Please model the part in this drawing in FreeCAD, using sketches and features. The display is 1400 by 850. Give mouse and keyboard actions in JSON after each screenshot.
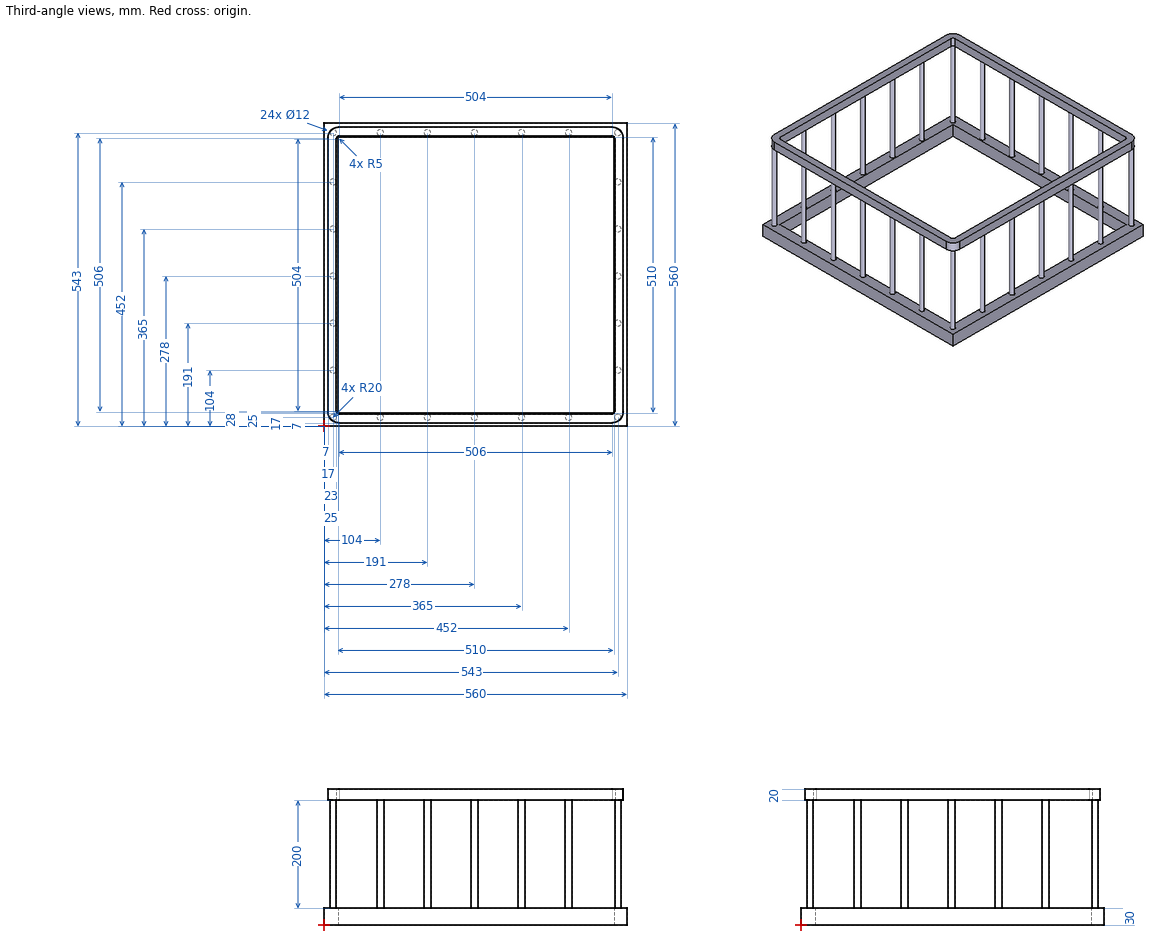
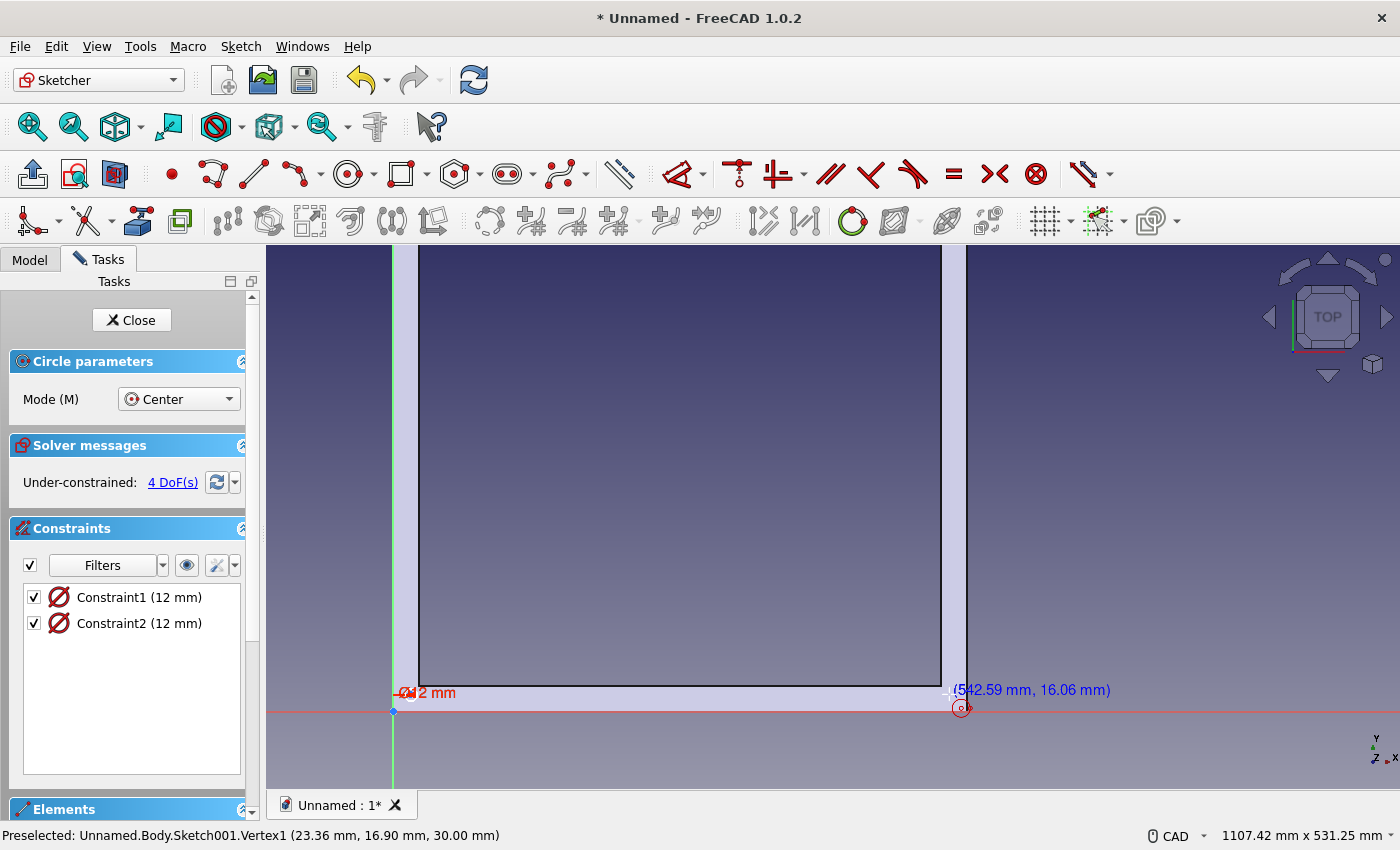
{"action": "left_click", "coordinate": [949, 694]}
{"action": "mouse_move", "coordinate": [953, 690]}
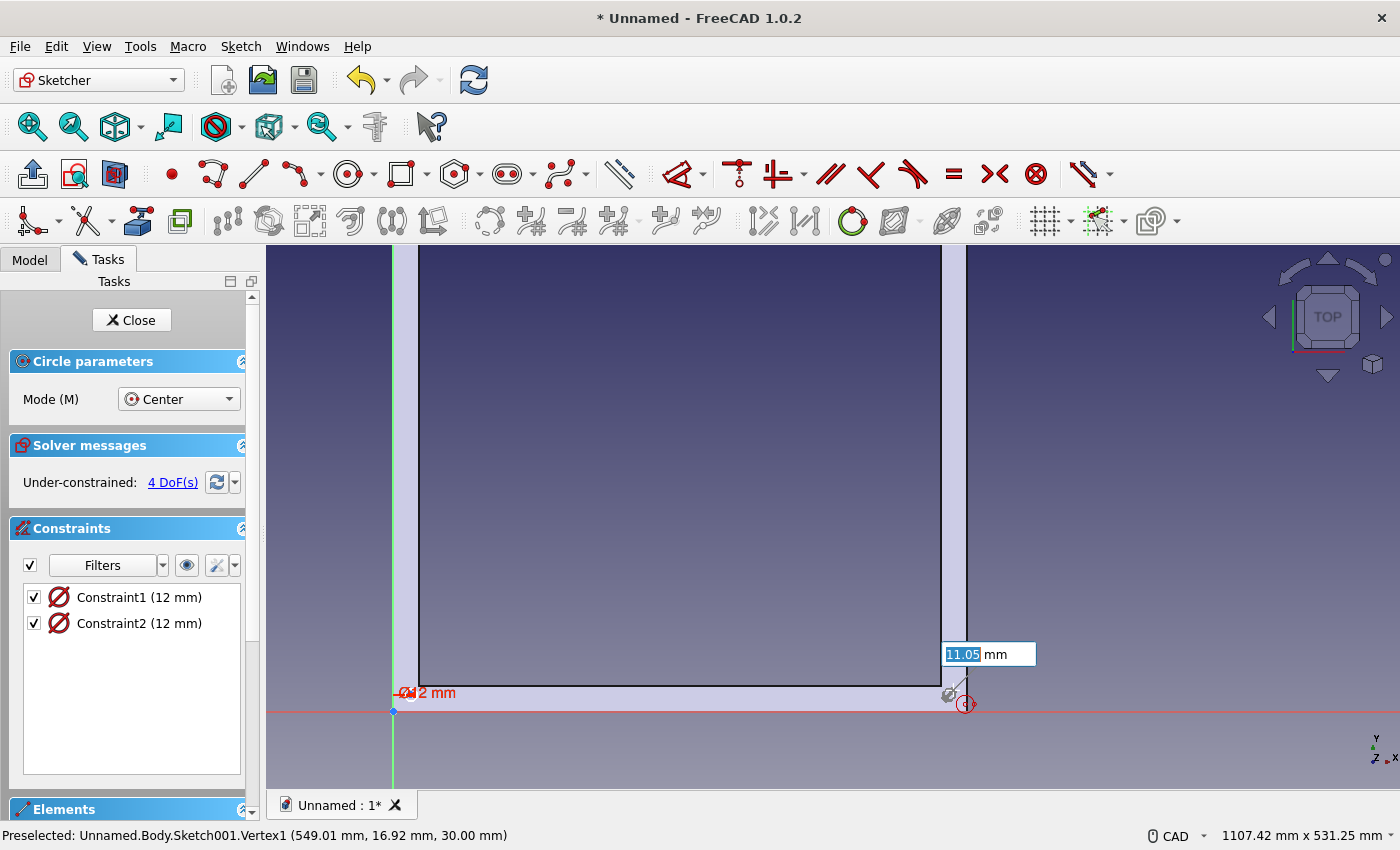
{"action": "type", "text": "12"}
{"action": "key", "text": "Return"}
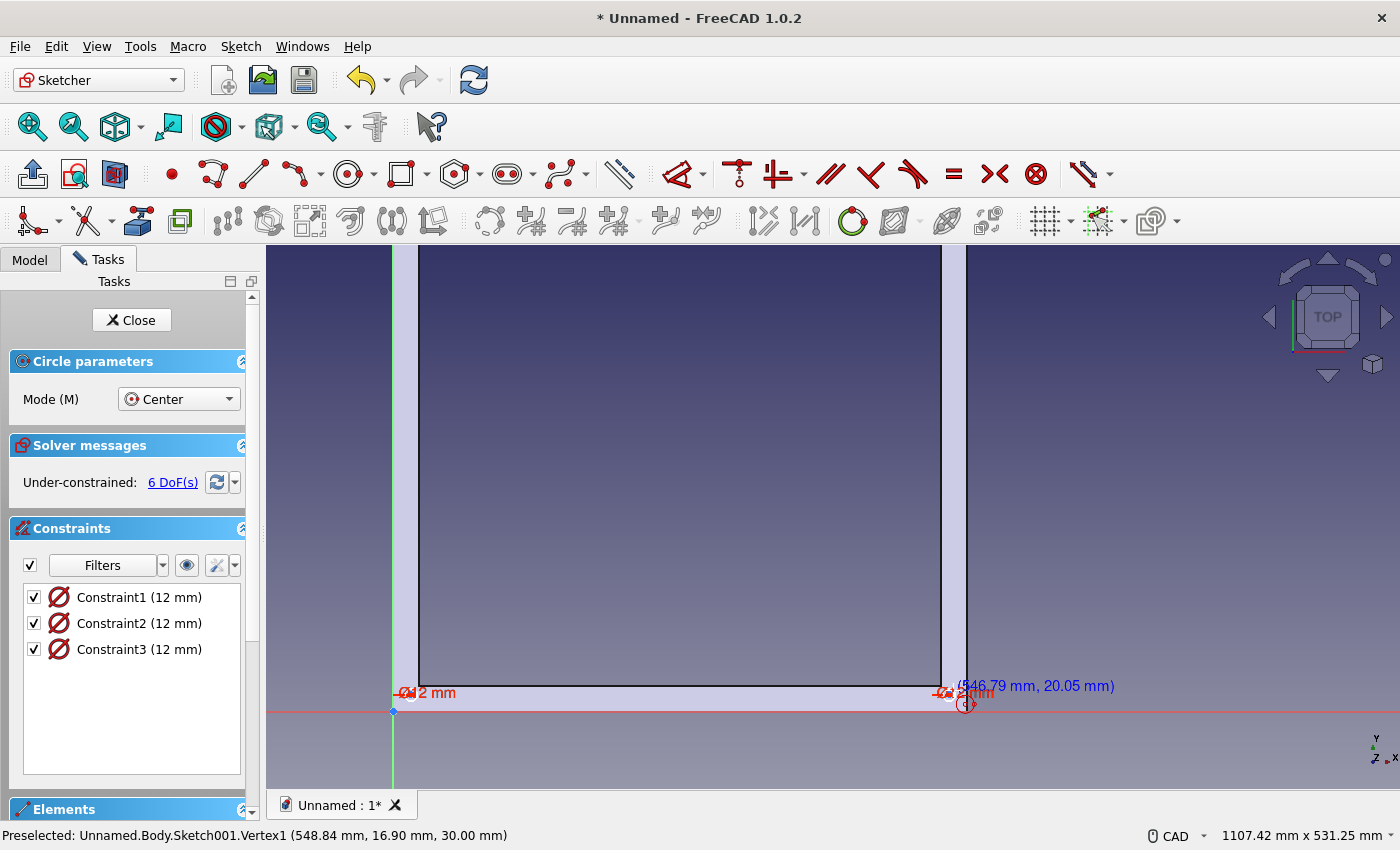
{"action": "scroll", "coordinate": [948, 693], "scroll_direction": "down", "scroll_amount": 2}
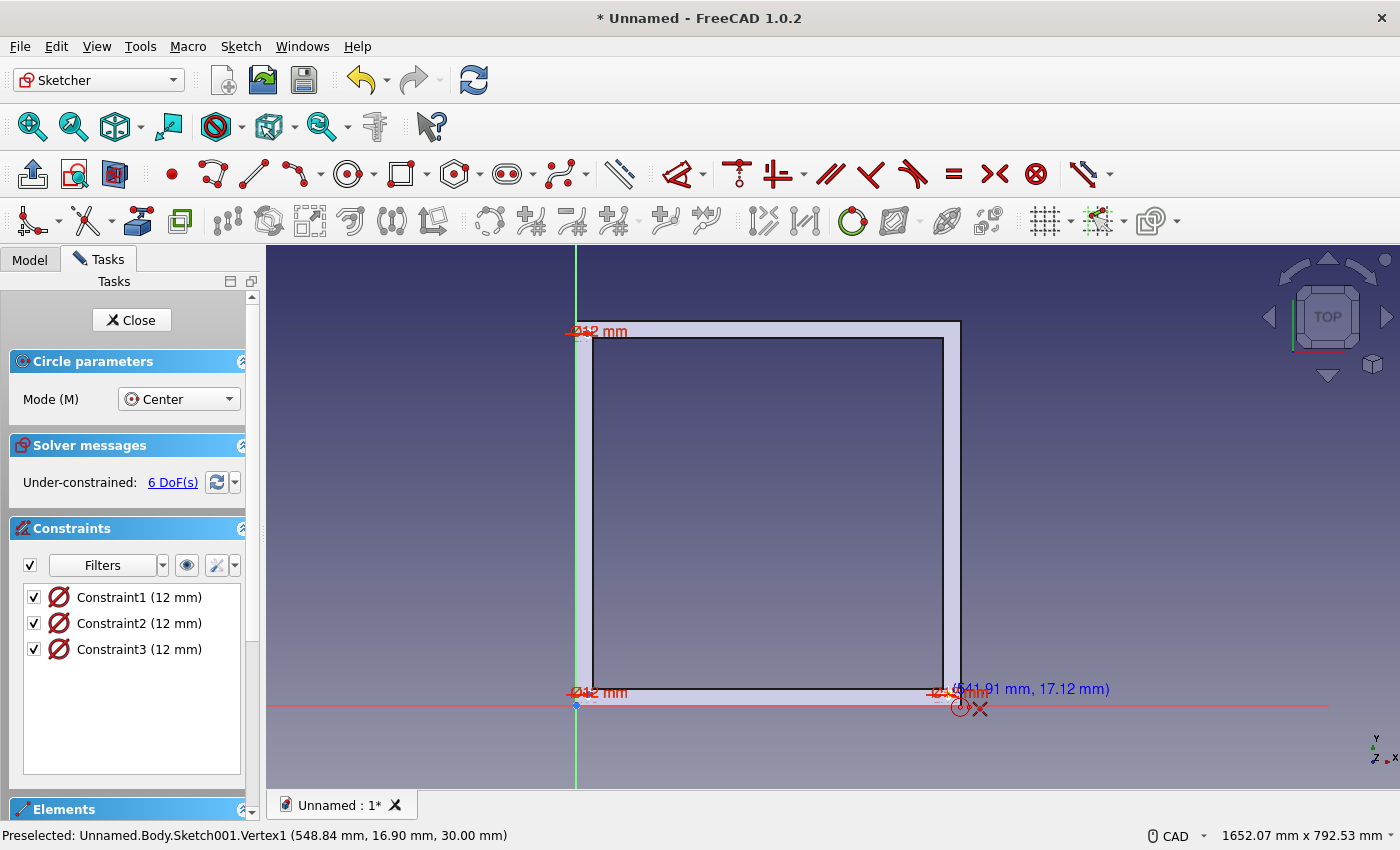
{"action": "scroll", "coordinate": [949, 333], "scroll_direction": "up", "scroll_amount": 9}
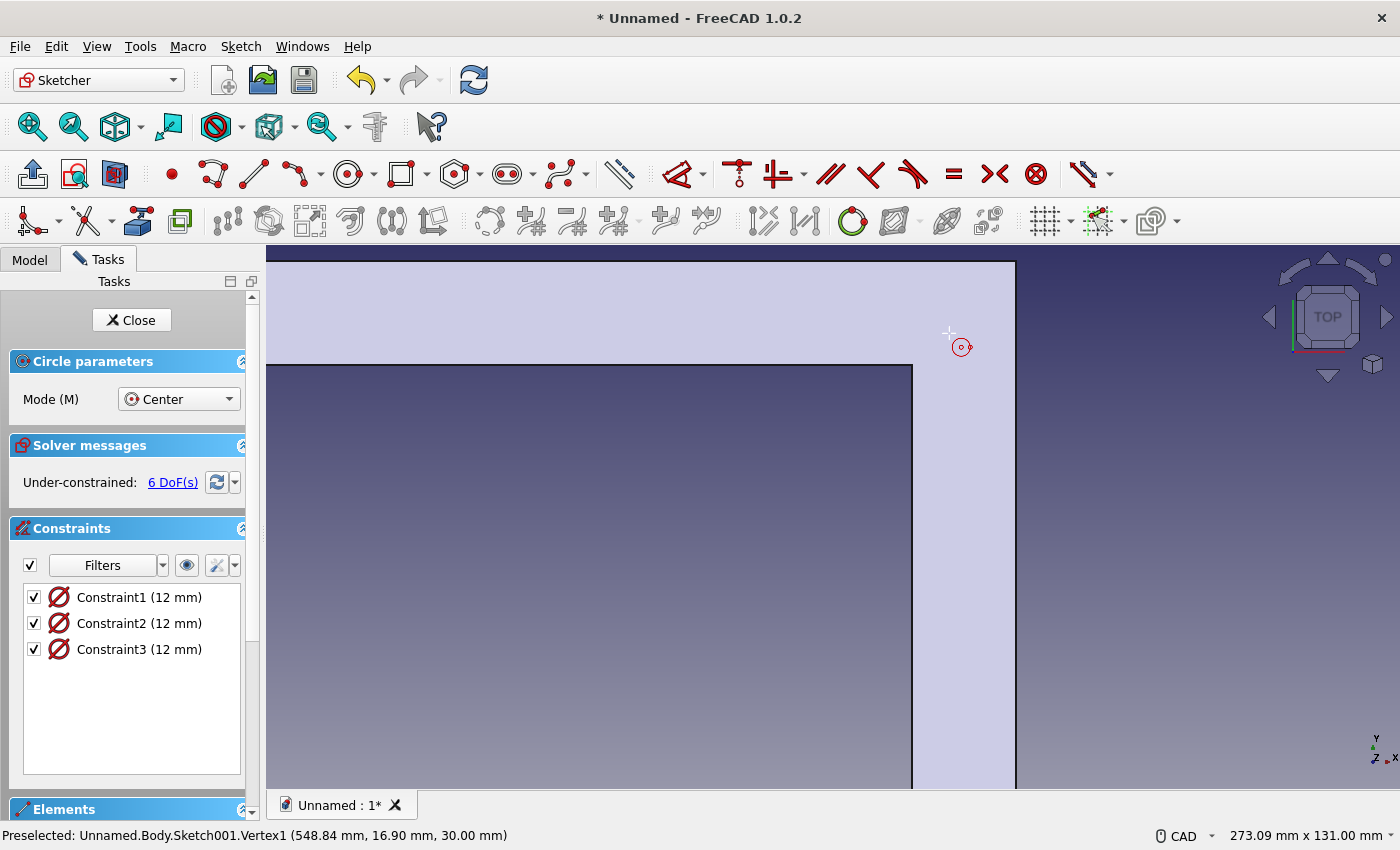
{"action": "scroll", "coordinate": [949, 333], "scroll_direction": "down", "scroll_amount": 9}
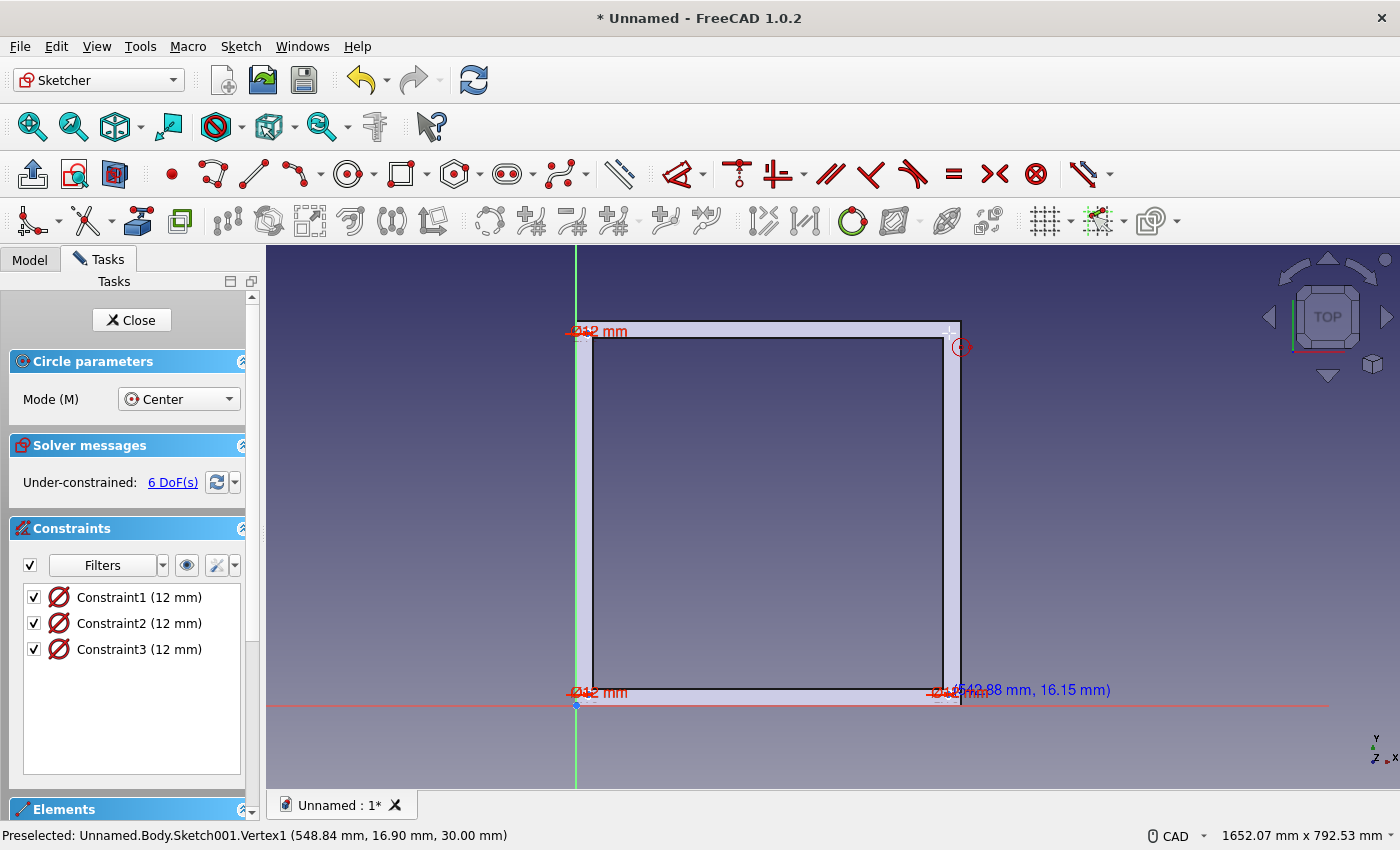
{"action": "left_click", "coordinate": [949, 333]}
{"action": "mouse_move", "coordinate": [952, 330]}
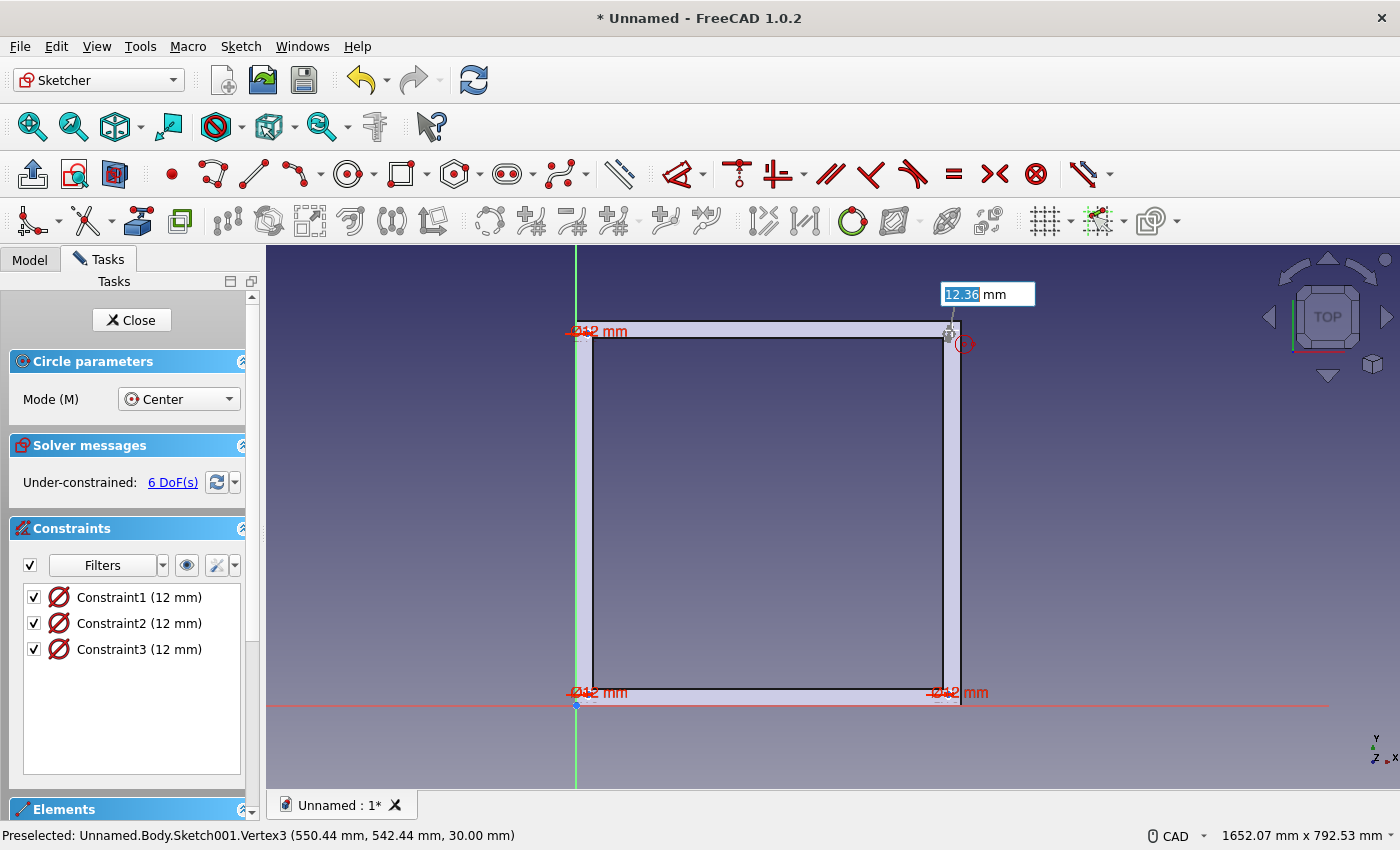
{"action": "type", "text": "12"}
{"action": "key", "text": "Return"}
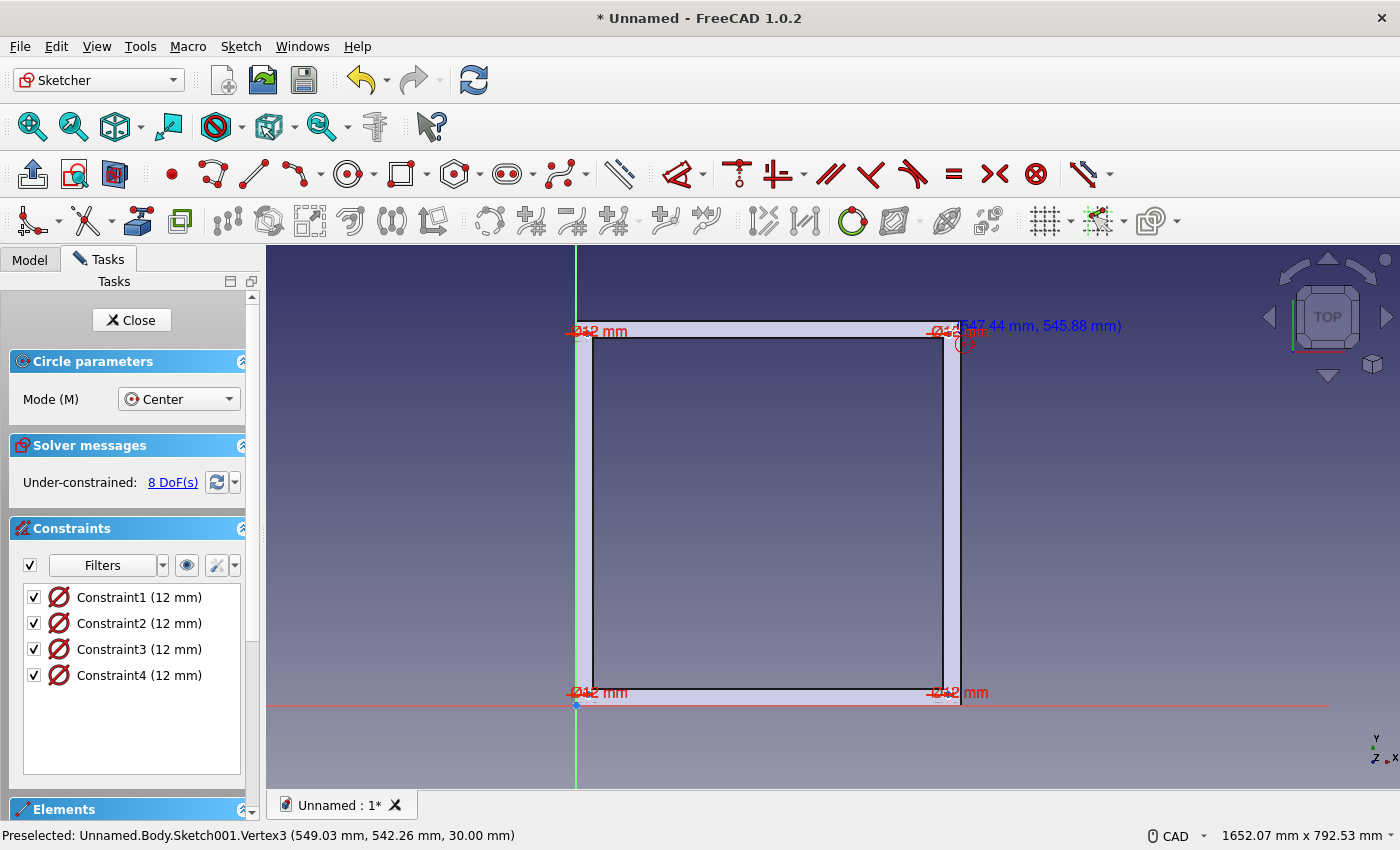
{"action": "scroll", "coordinate": [648, 333], "scroll_direction": "up", "scroll_amount": 9}